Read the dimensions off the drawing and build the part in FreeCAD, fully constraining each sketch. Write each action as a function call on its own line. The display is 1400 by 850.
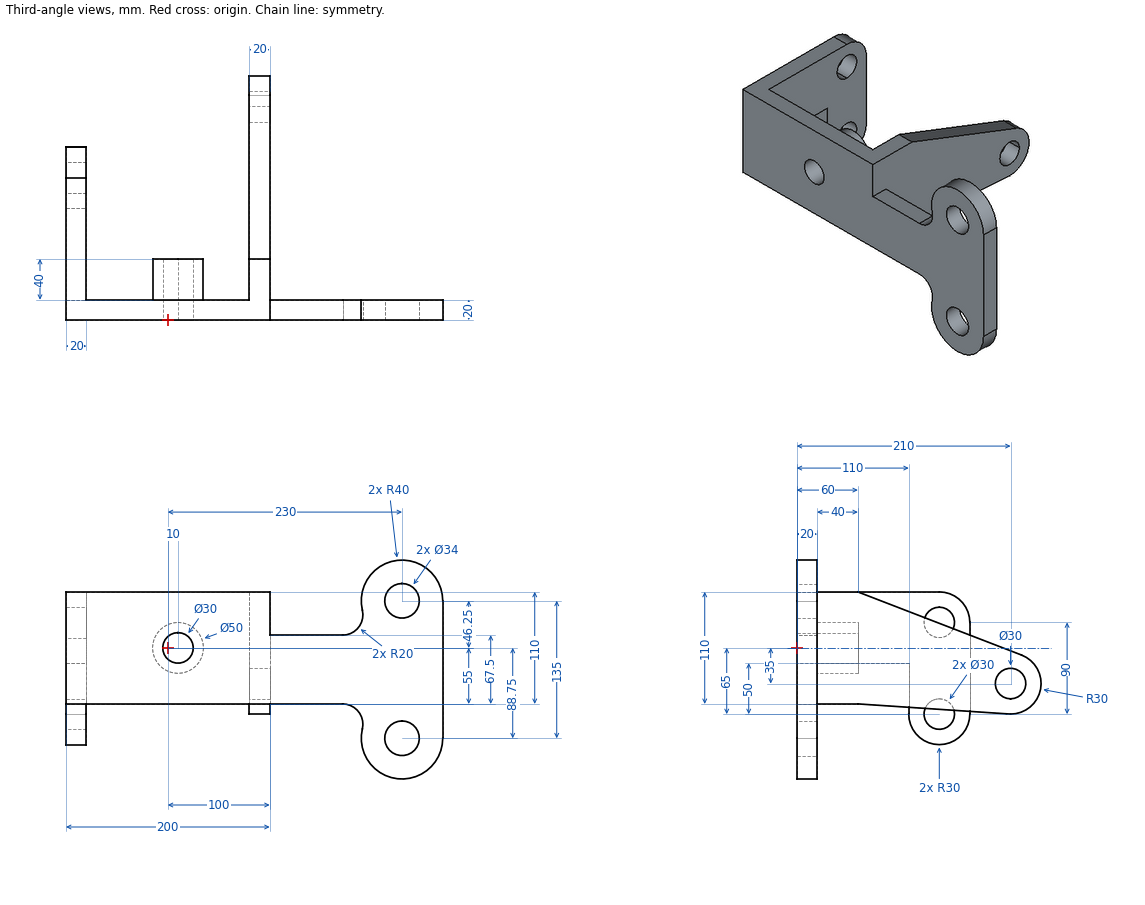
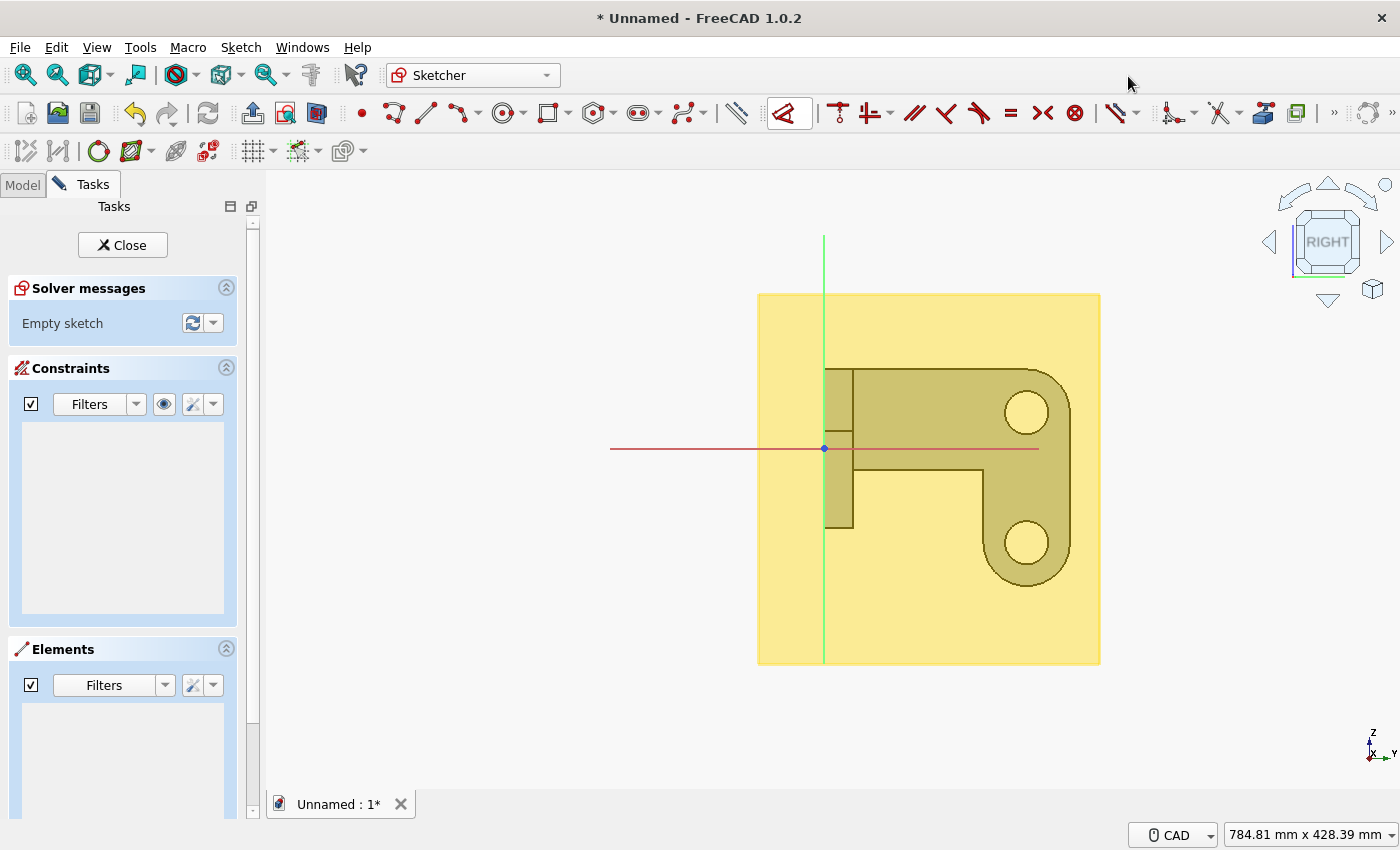
scroll(1235, 427, up, 3)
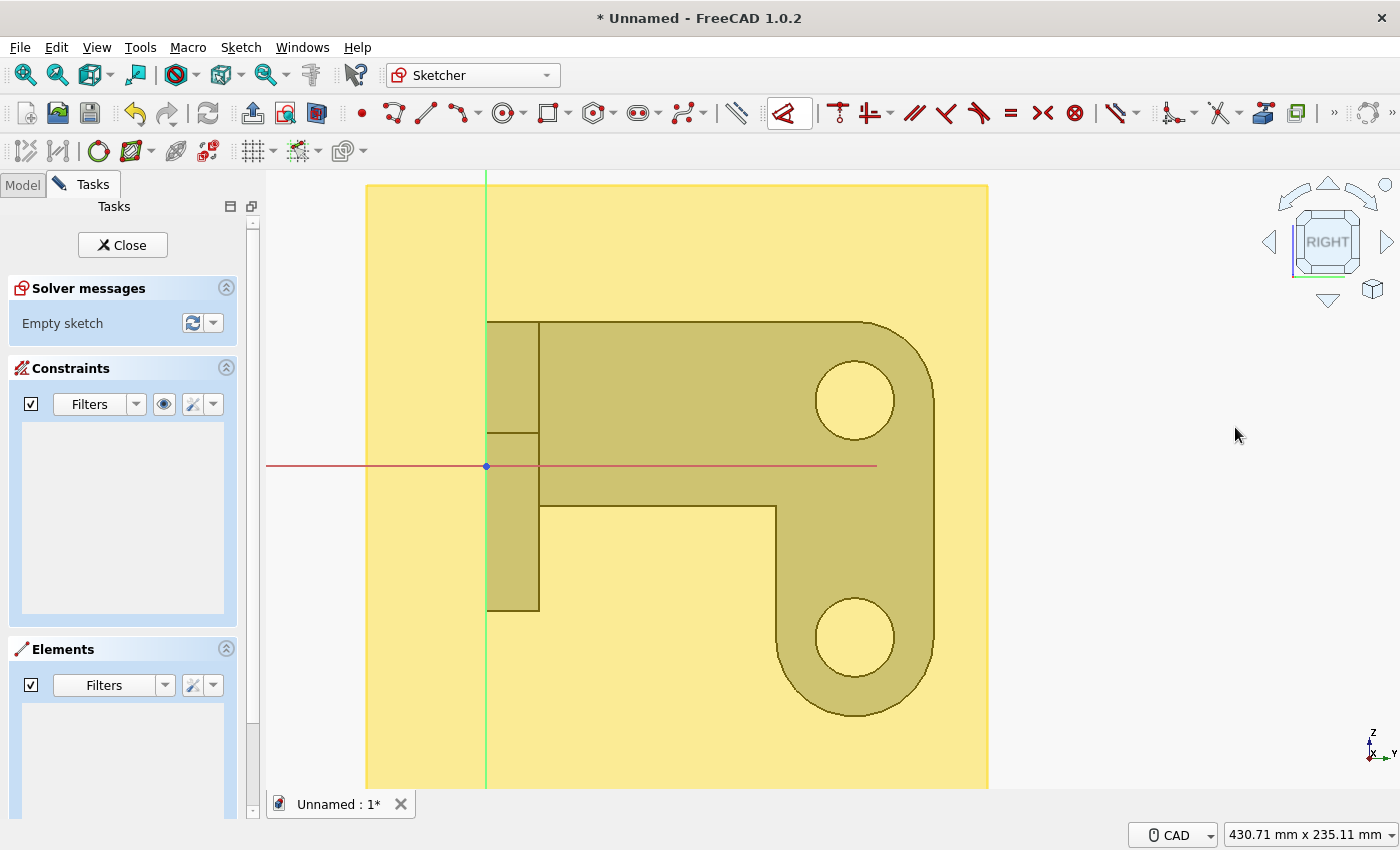
key(g)
key(m)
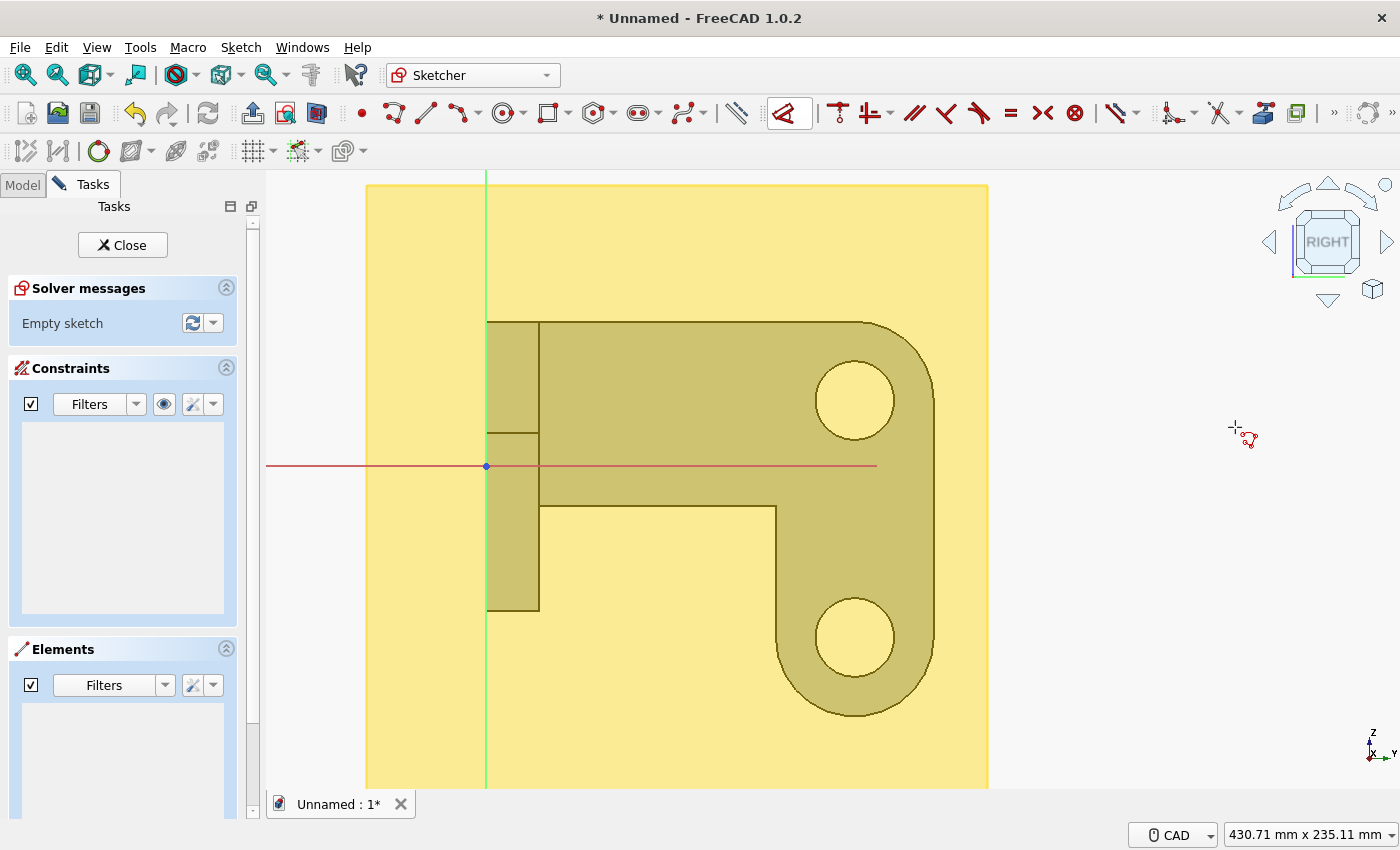
click(1067, 485)
click(644, 322)
click(539, 322)
click(539, 611)
click(644, 611)
click(1039, 638)
right_click(1039, 638)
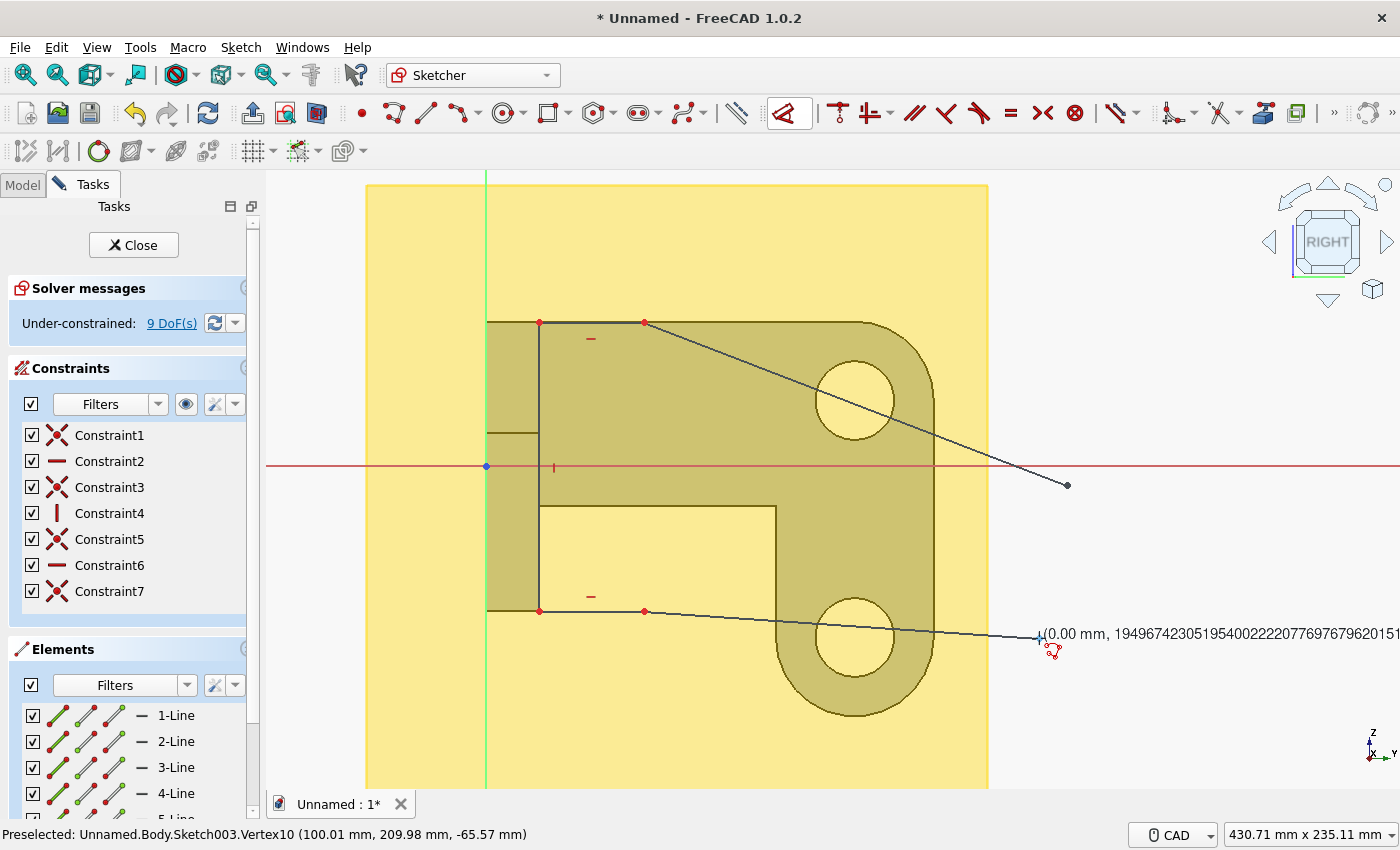
click(458, 114)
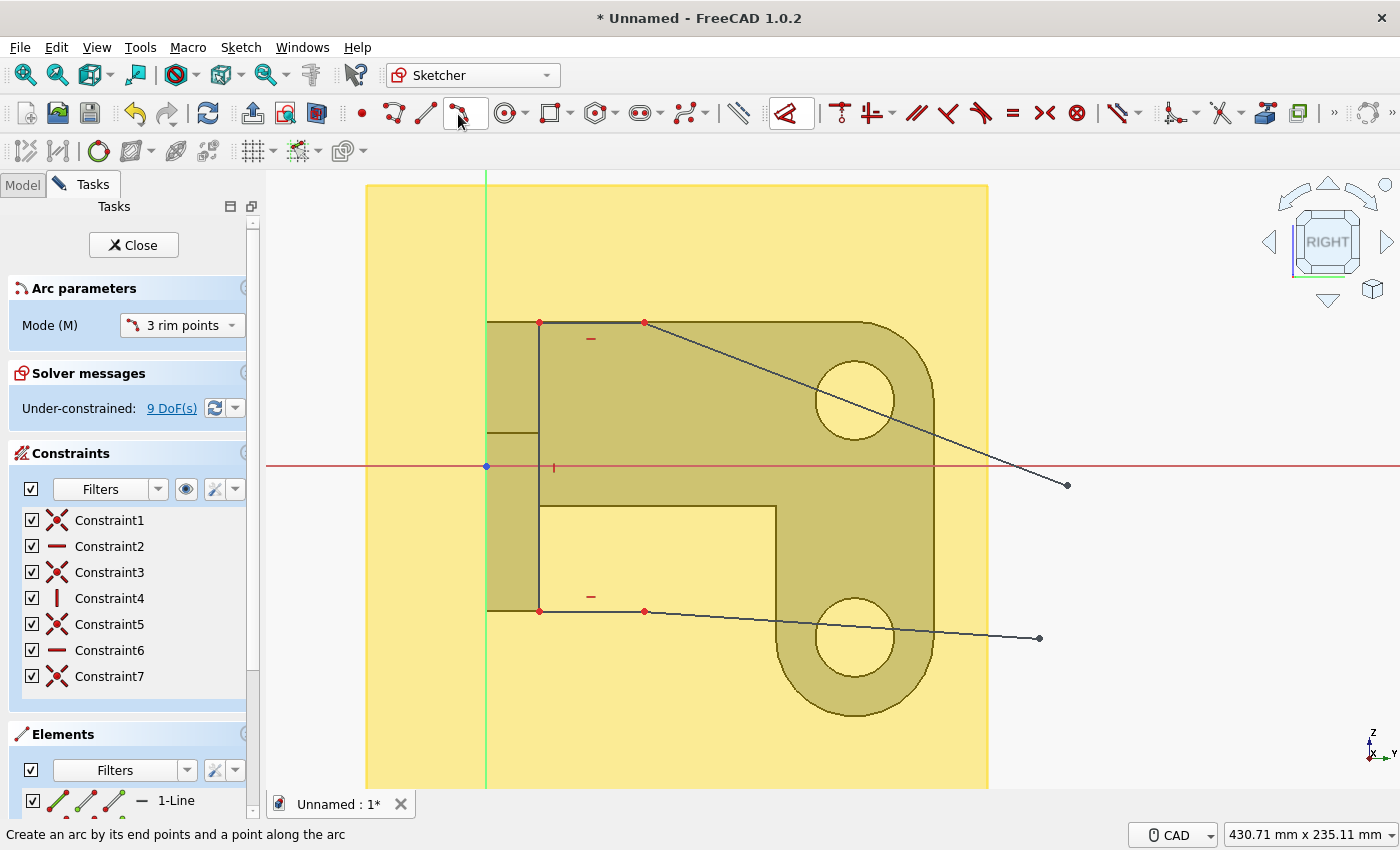
click(1039, 639)
click(1067, 486)
click(1117, 573)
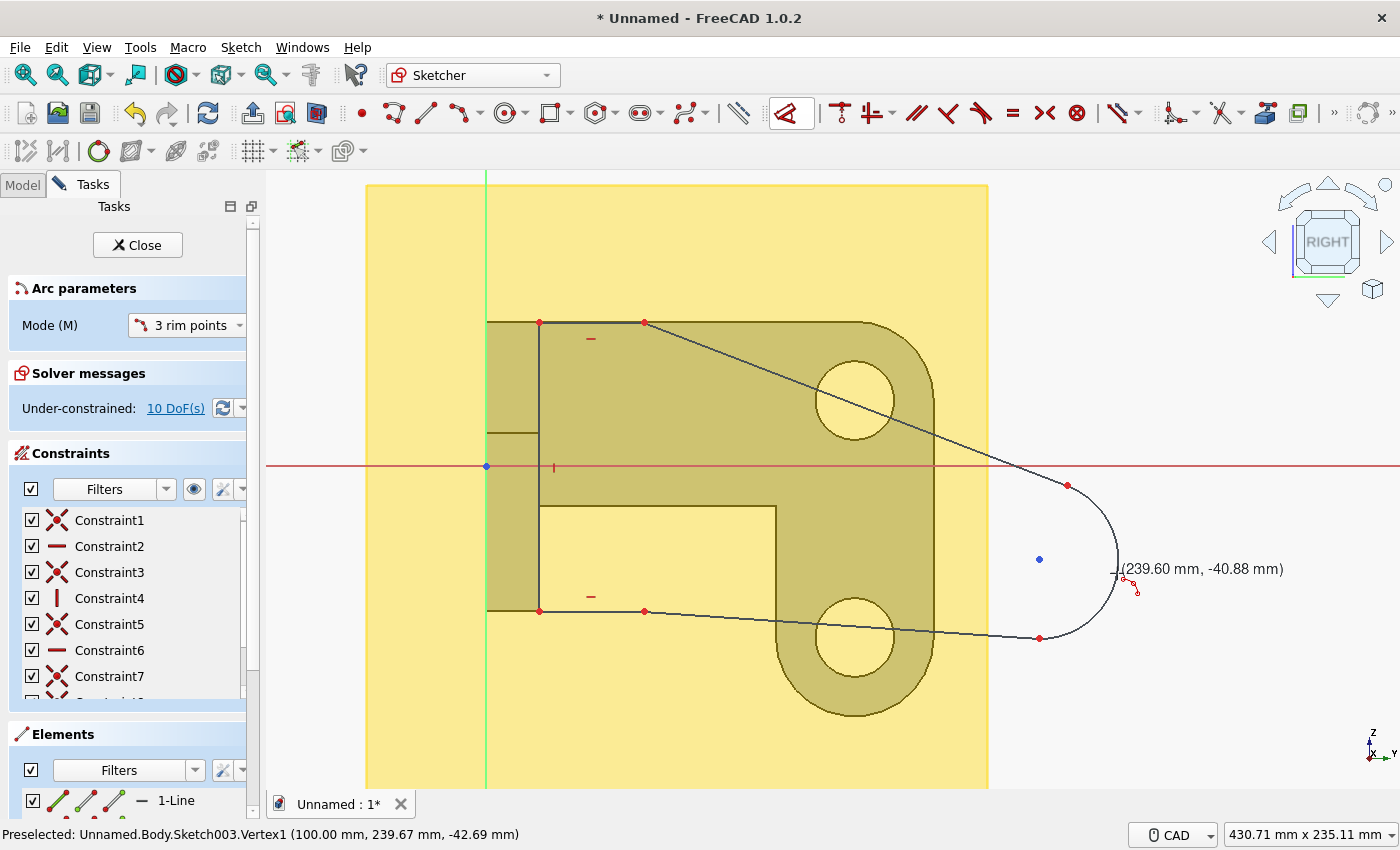
key(g)
key(c)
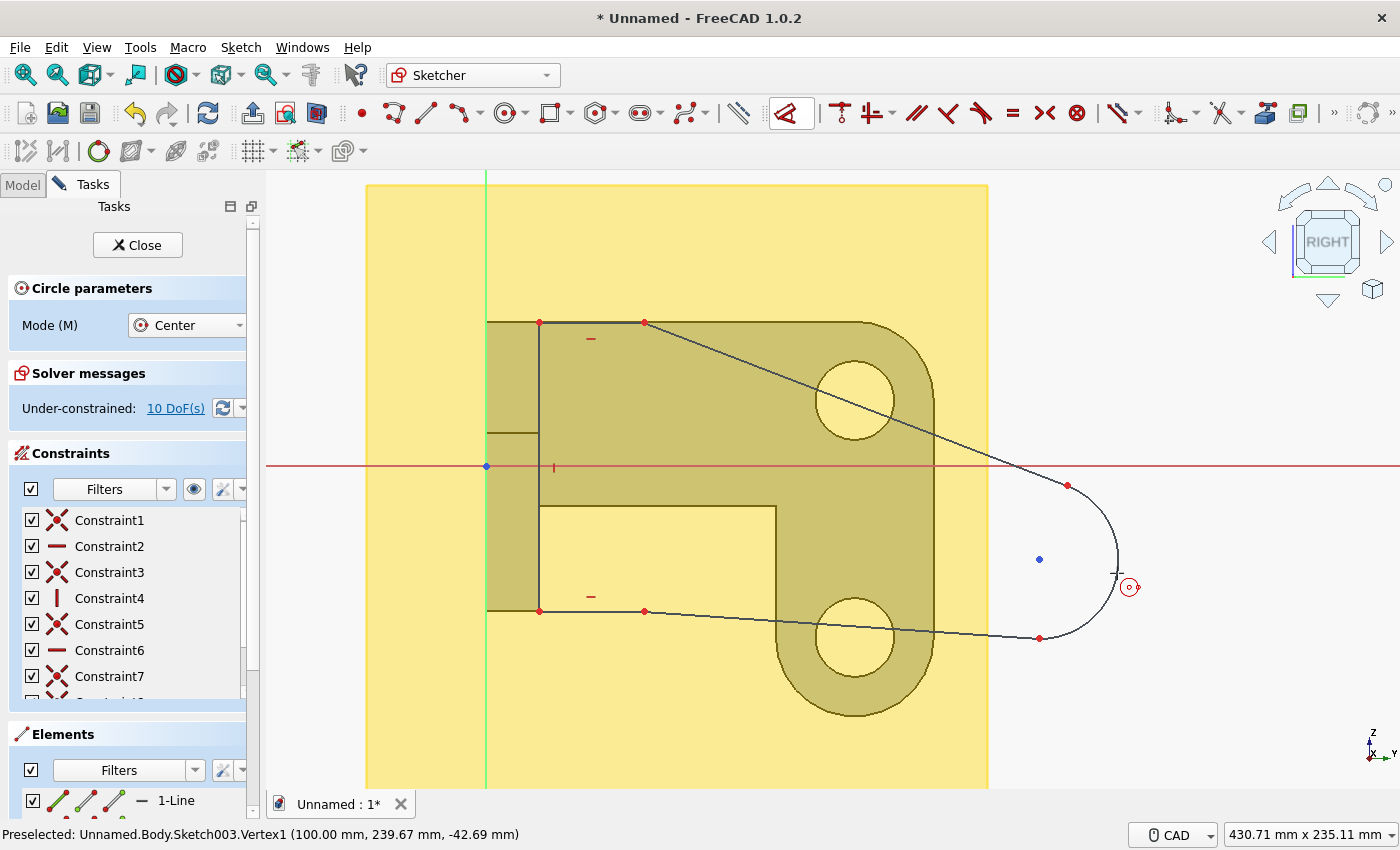
click(1039, 559)
click(1067, 531)
key(Escape)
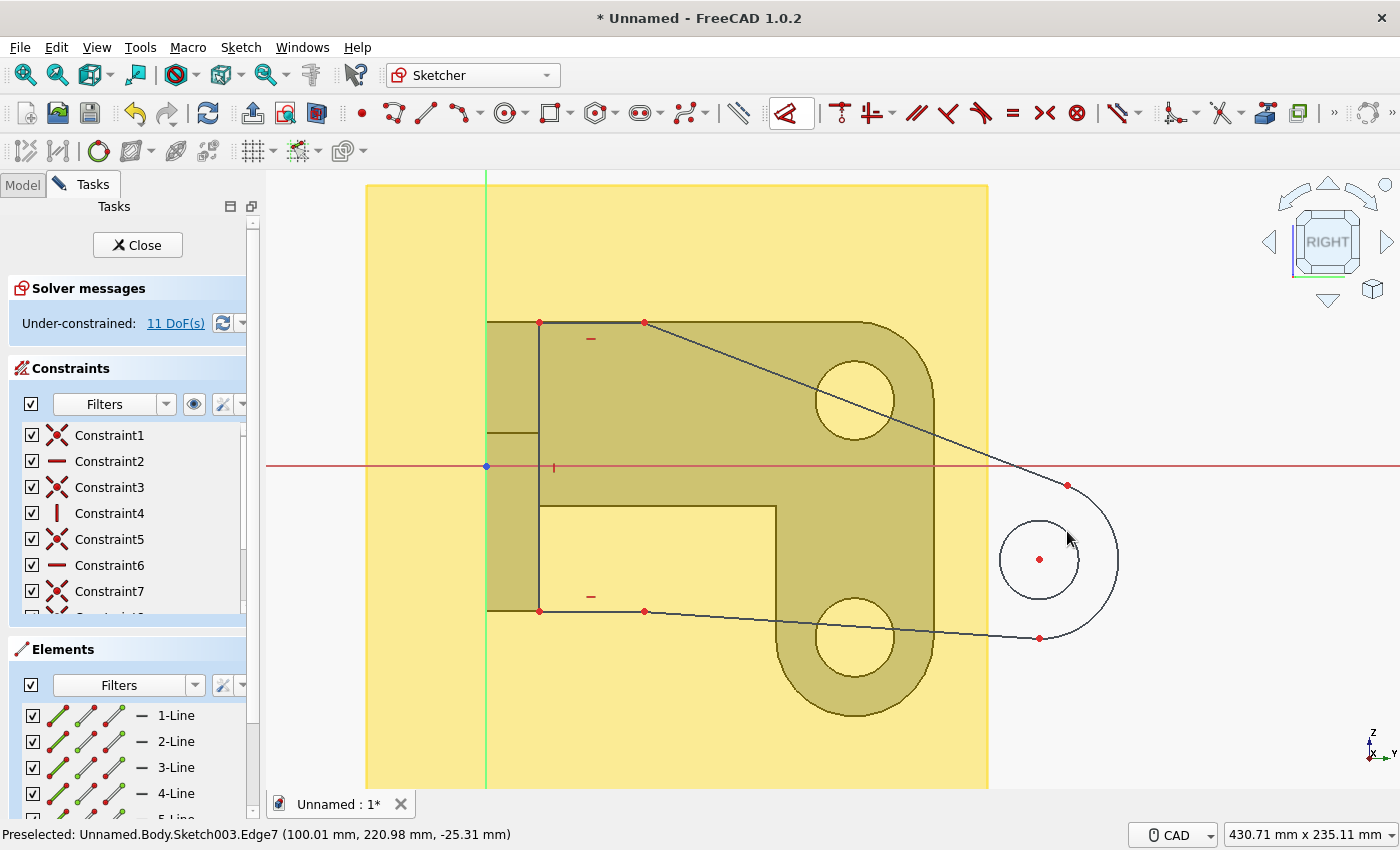
click(940, 437)